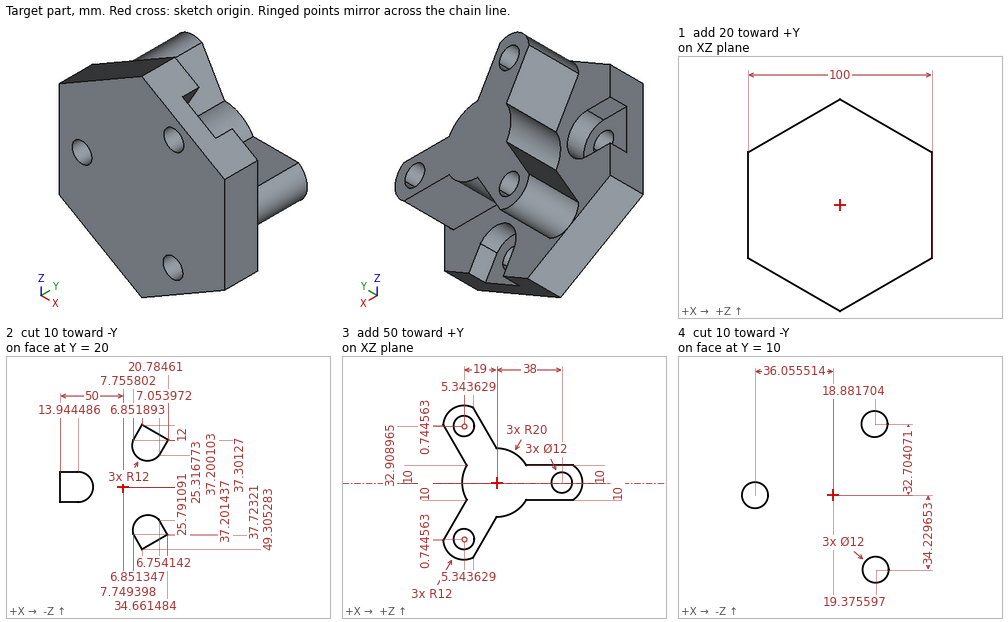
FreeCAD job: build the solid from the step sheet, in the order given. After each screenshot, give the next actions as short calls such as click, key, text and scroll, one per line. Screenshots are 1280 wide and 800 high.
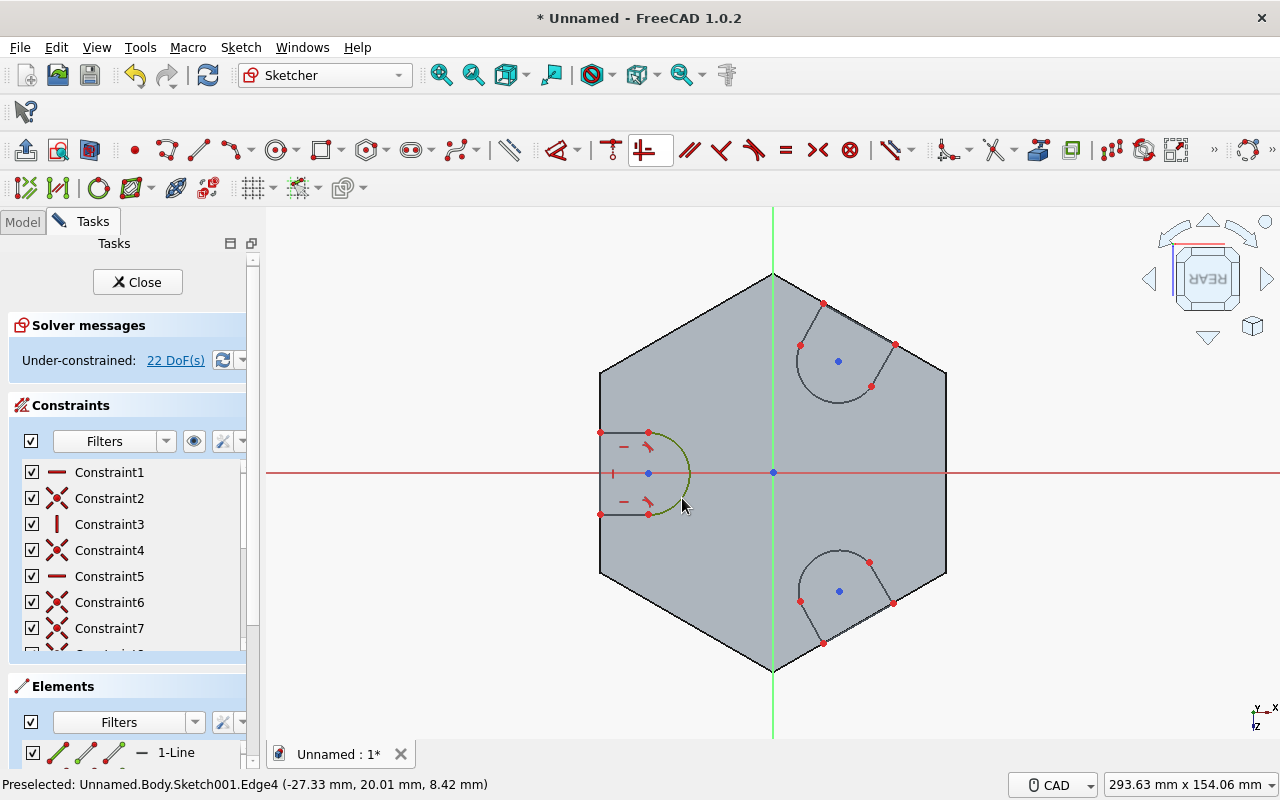
click(802, 380)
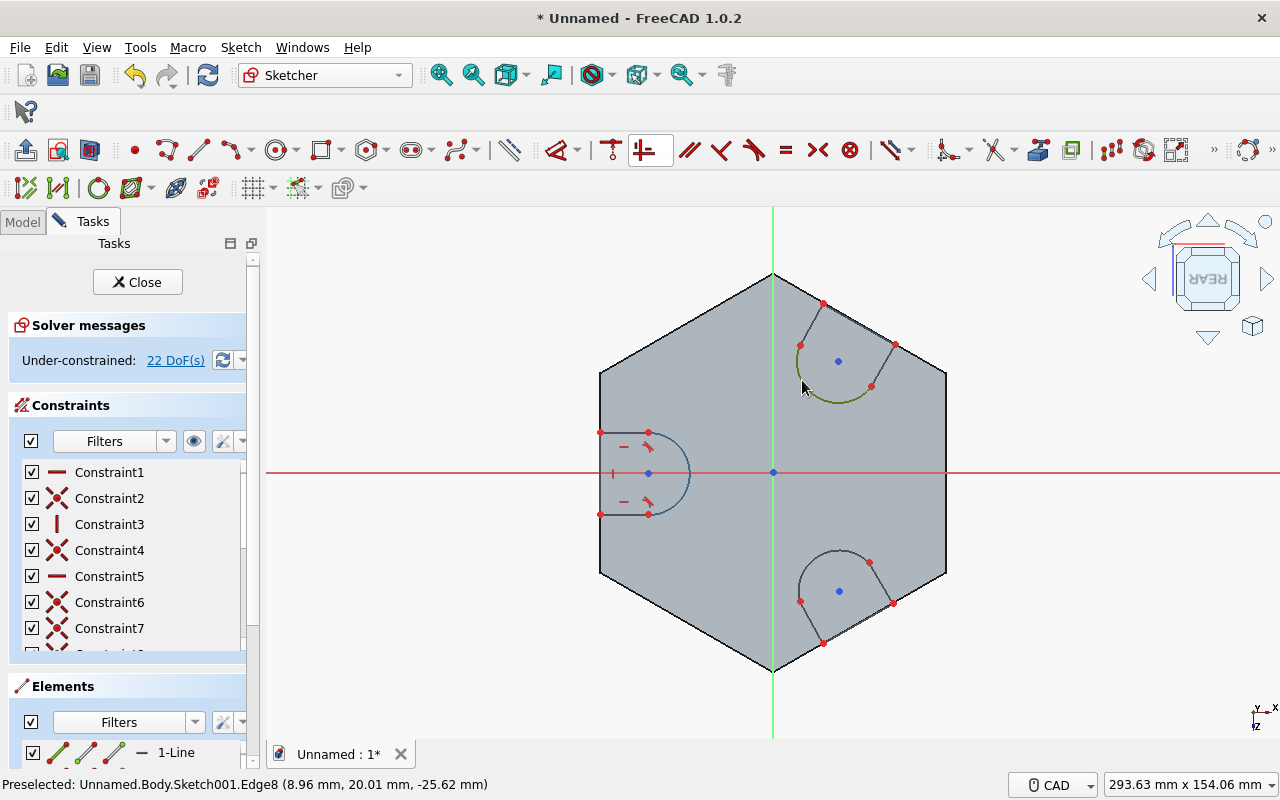
click(840, 550)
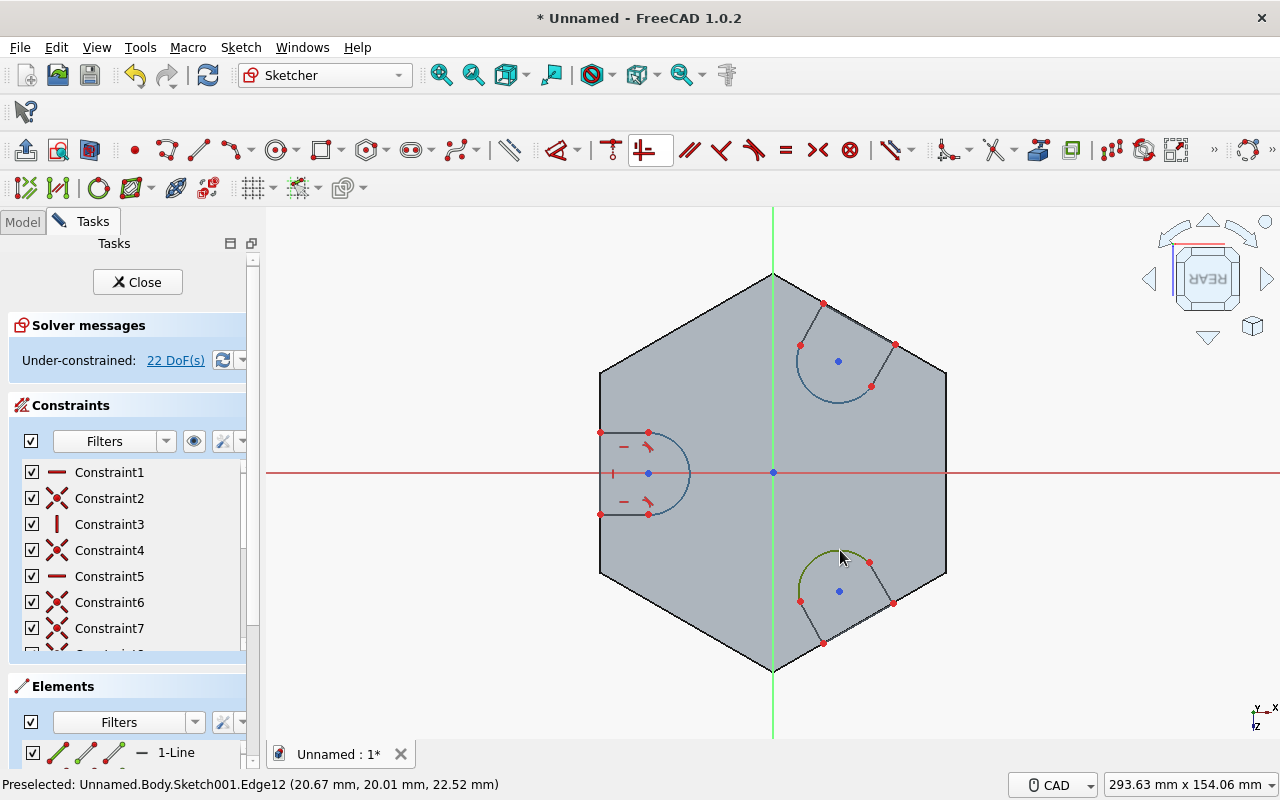
click(786, 150)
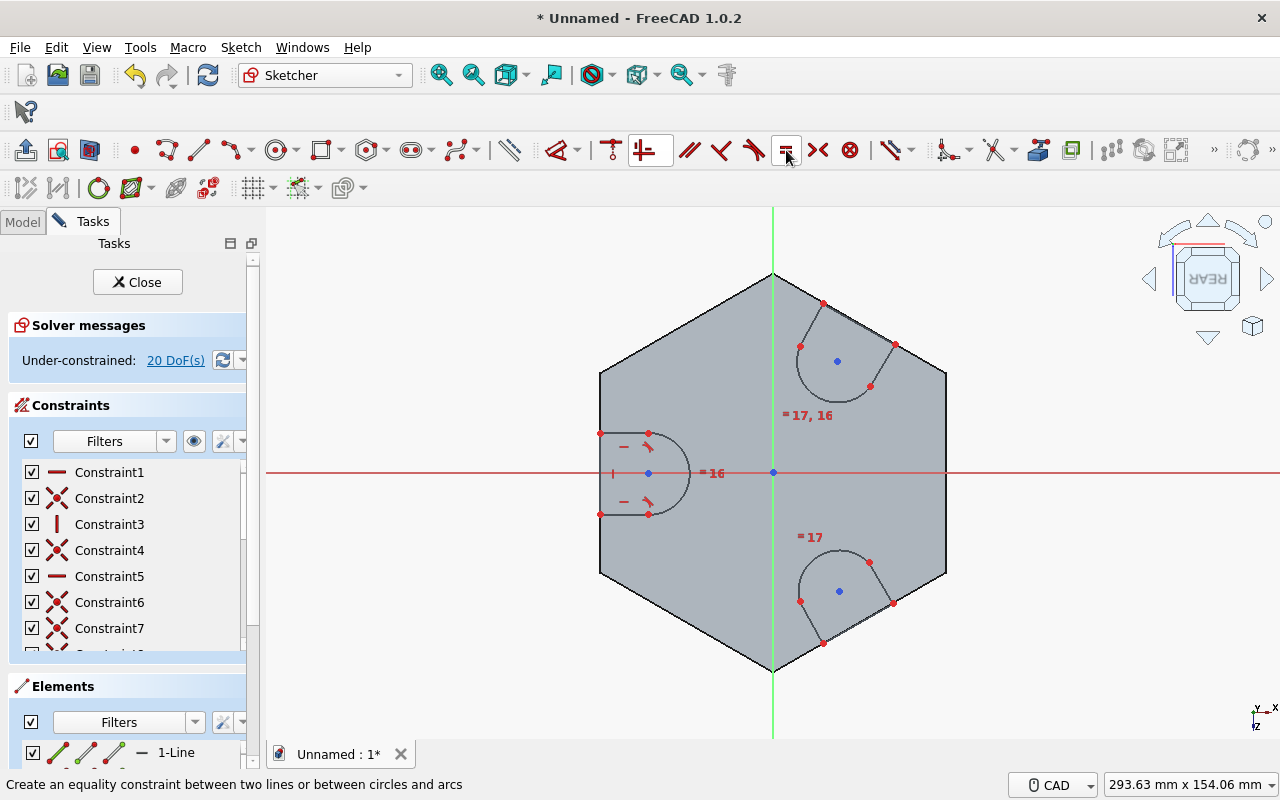
click(649, 474)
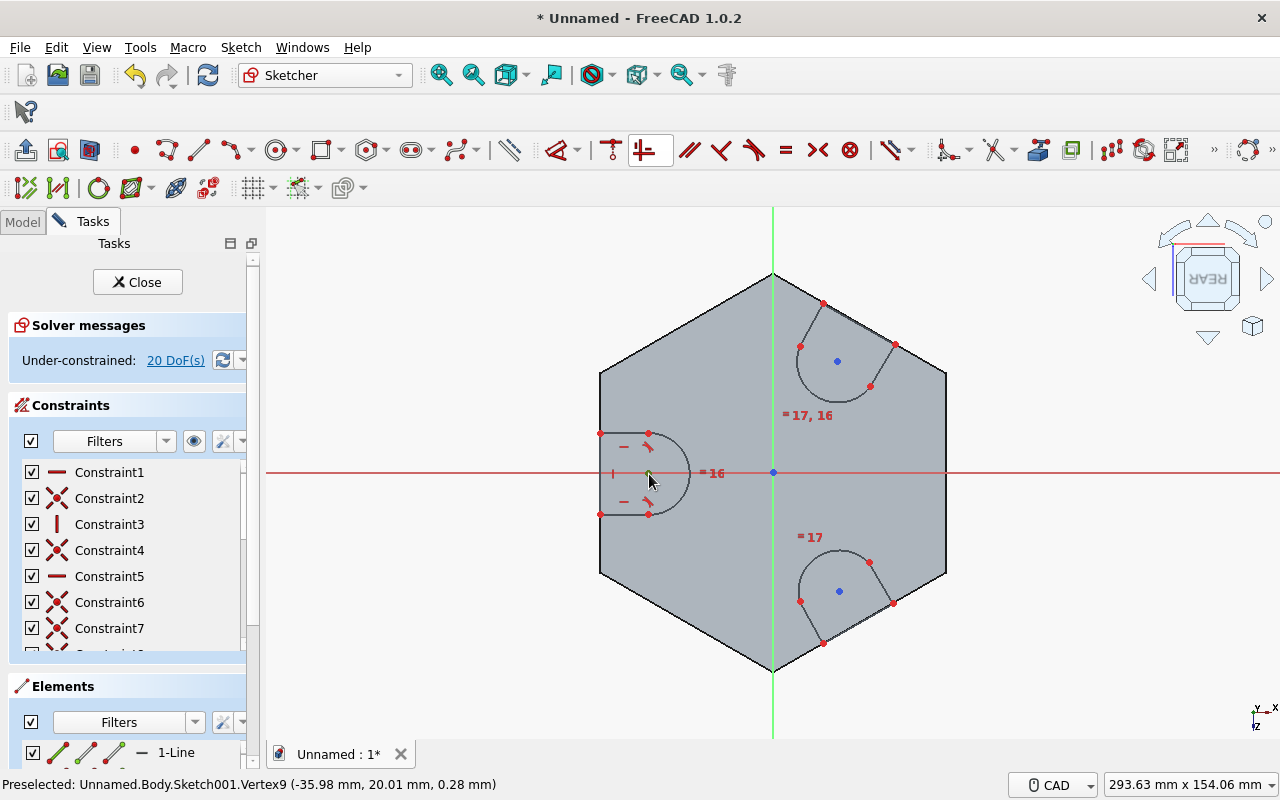
click(353, 473)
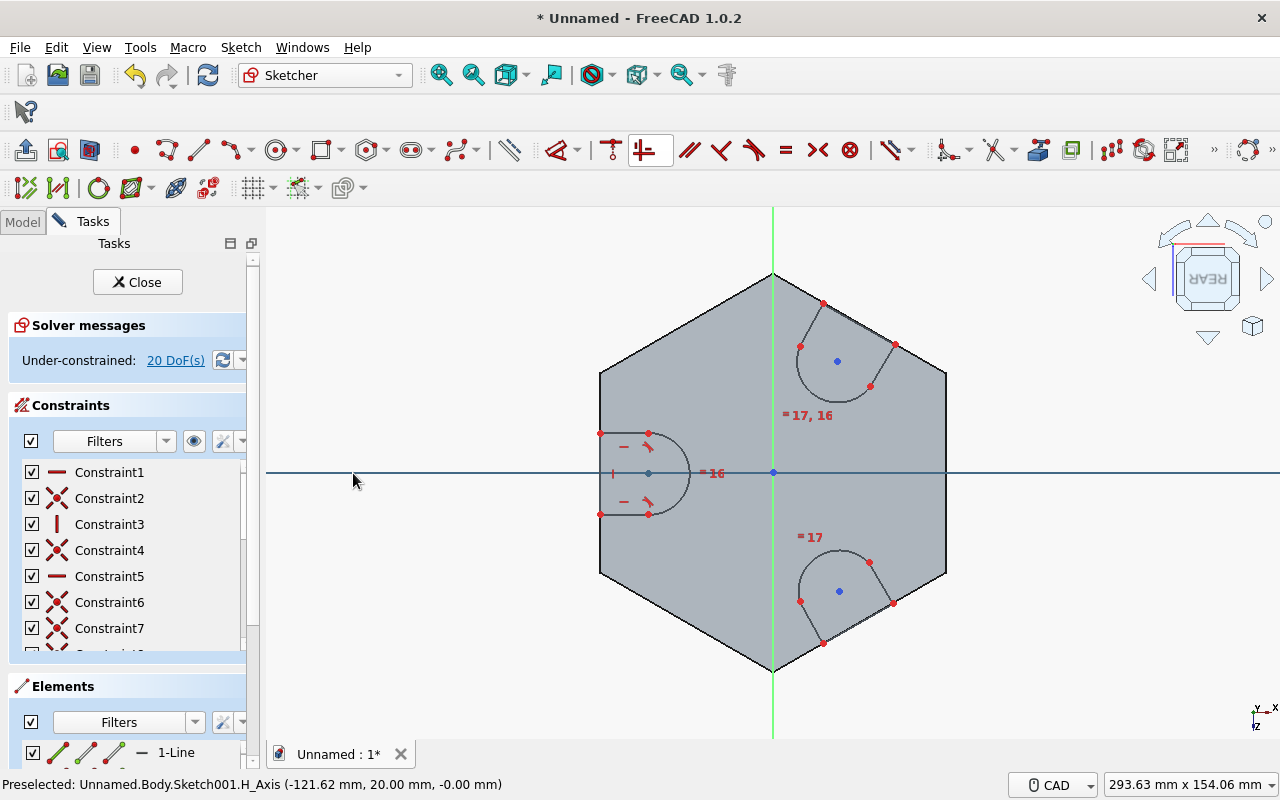
key(c)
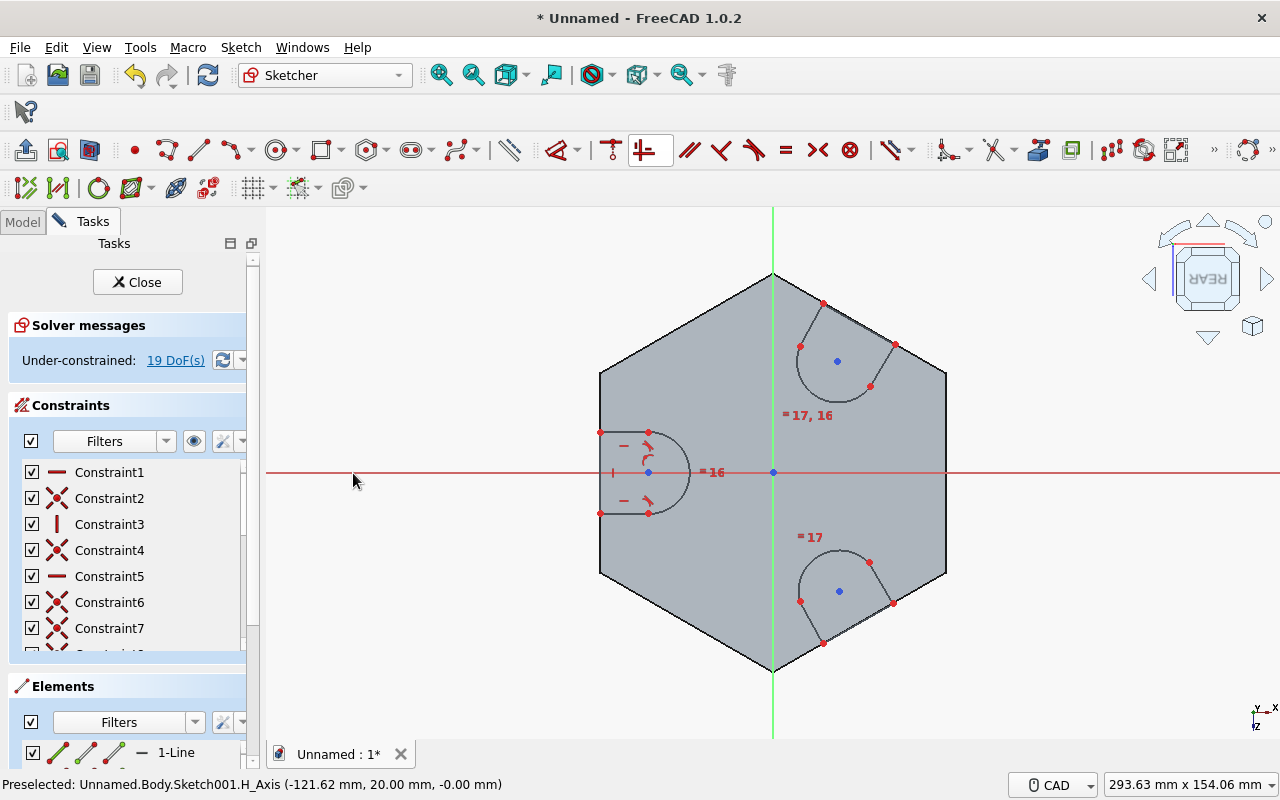
click(556, 150)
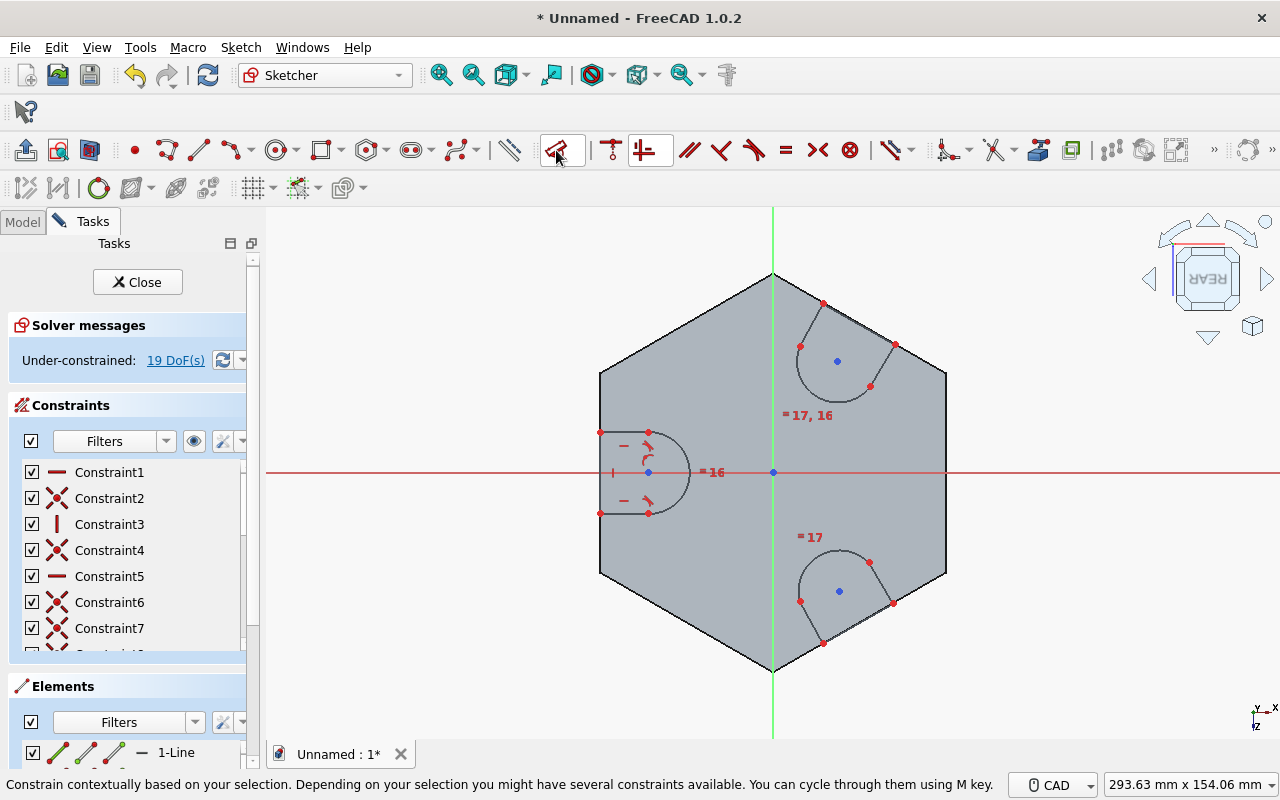
click(682, 497)
click(708, 516)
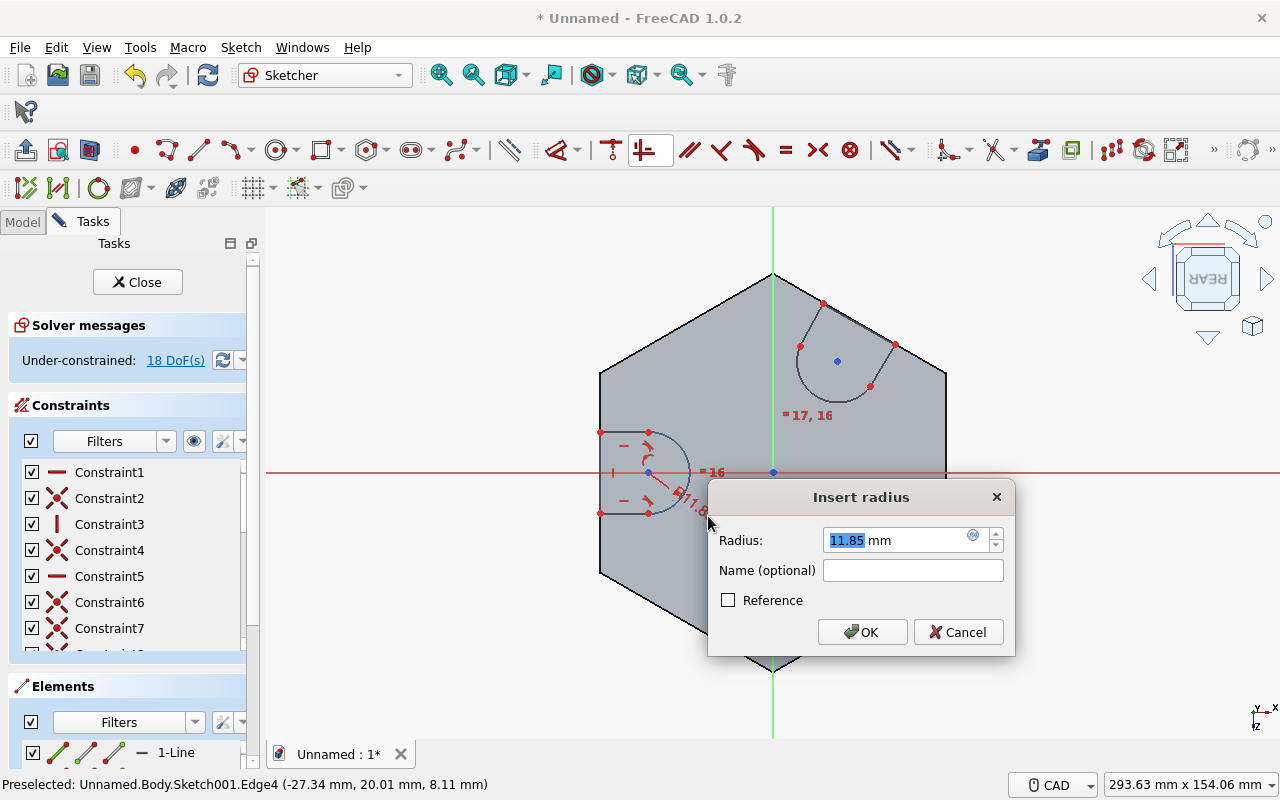
text(12)
key(Return)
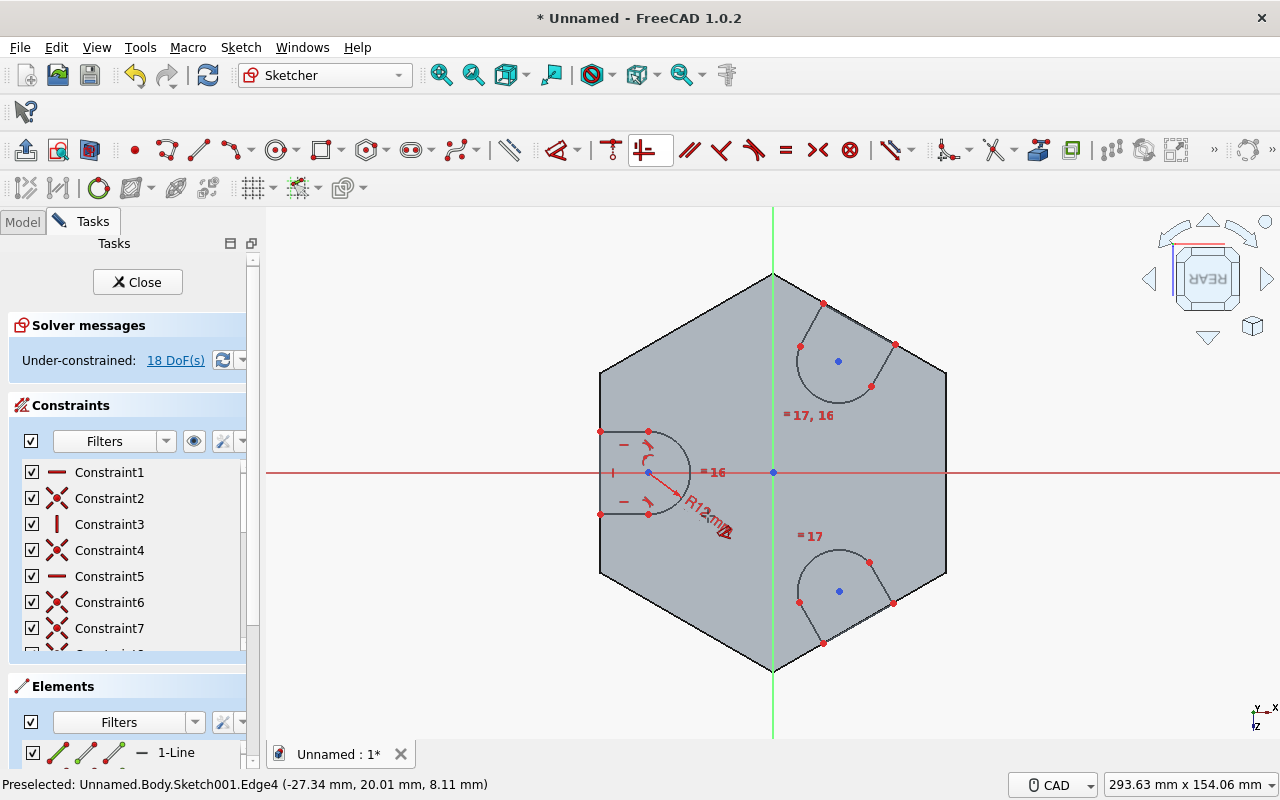
click(600, 432)
click(686, 398)